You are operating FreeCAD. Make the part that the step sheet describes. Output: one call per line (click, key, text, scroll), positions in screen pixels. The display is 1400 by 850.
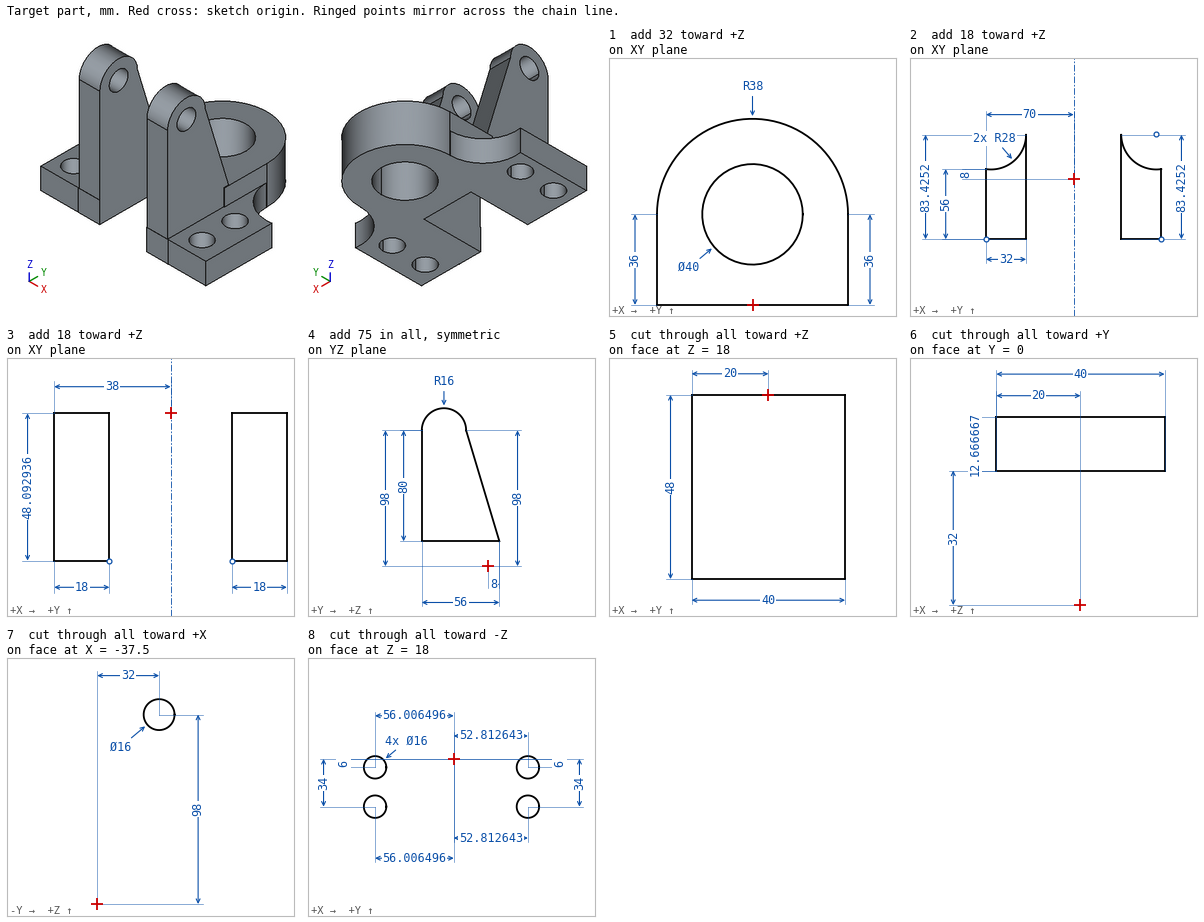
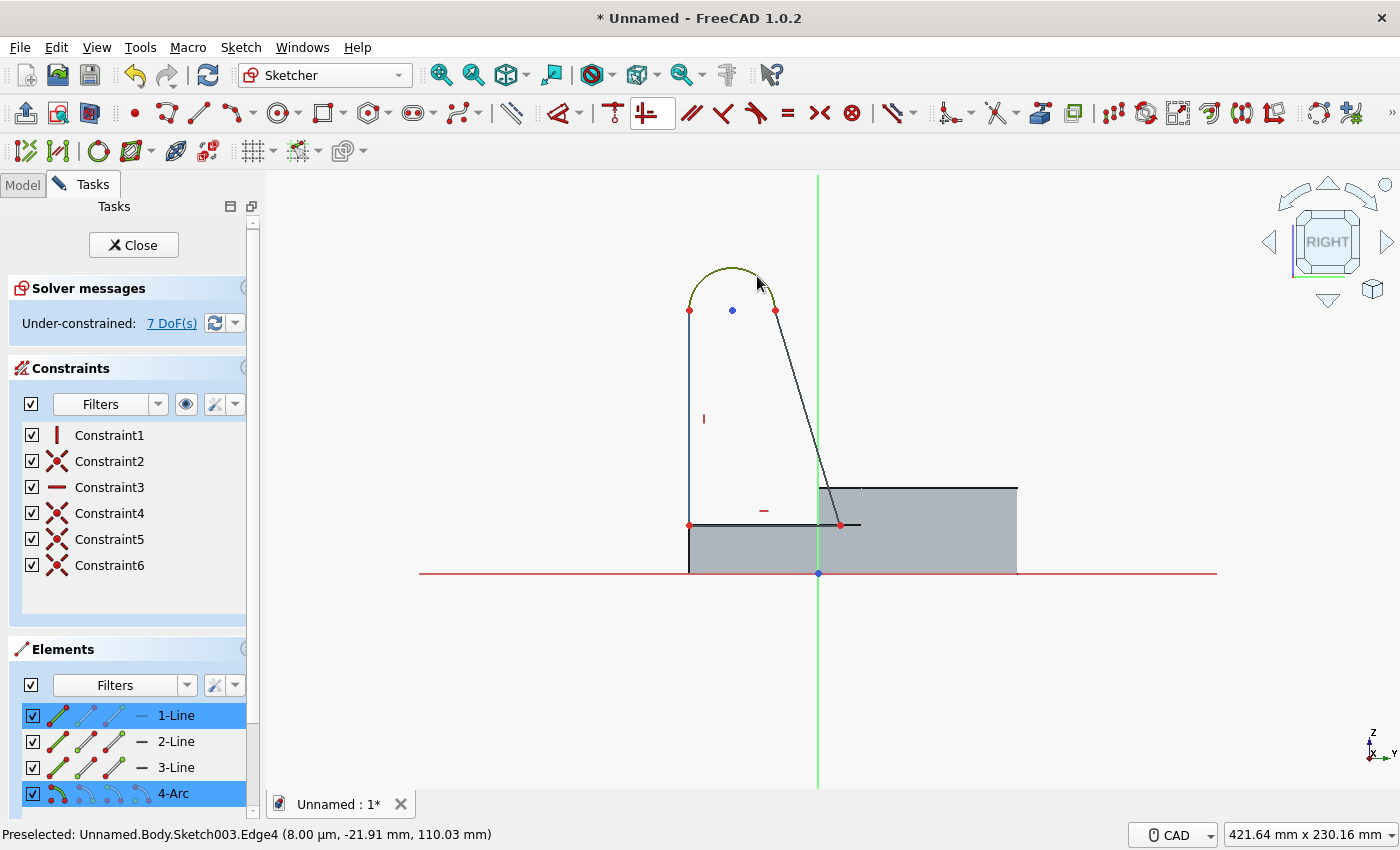
click(756, 114)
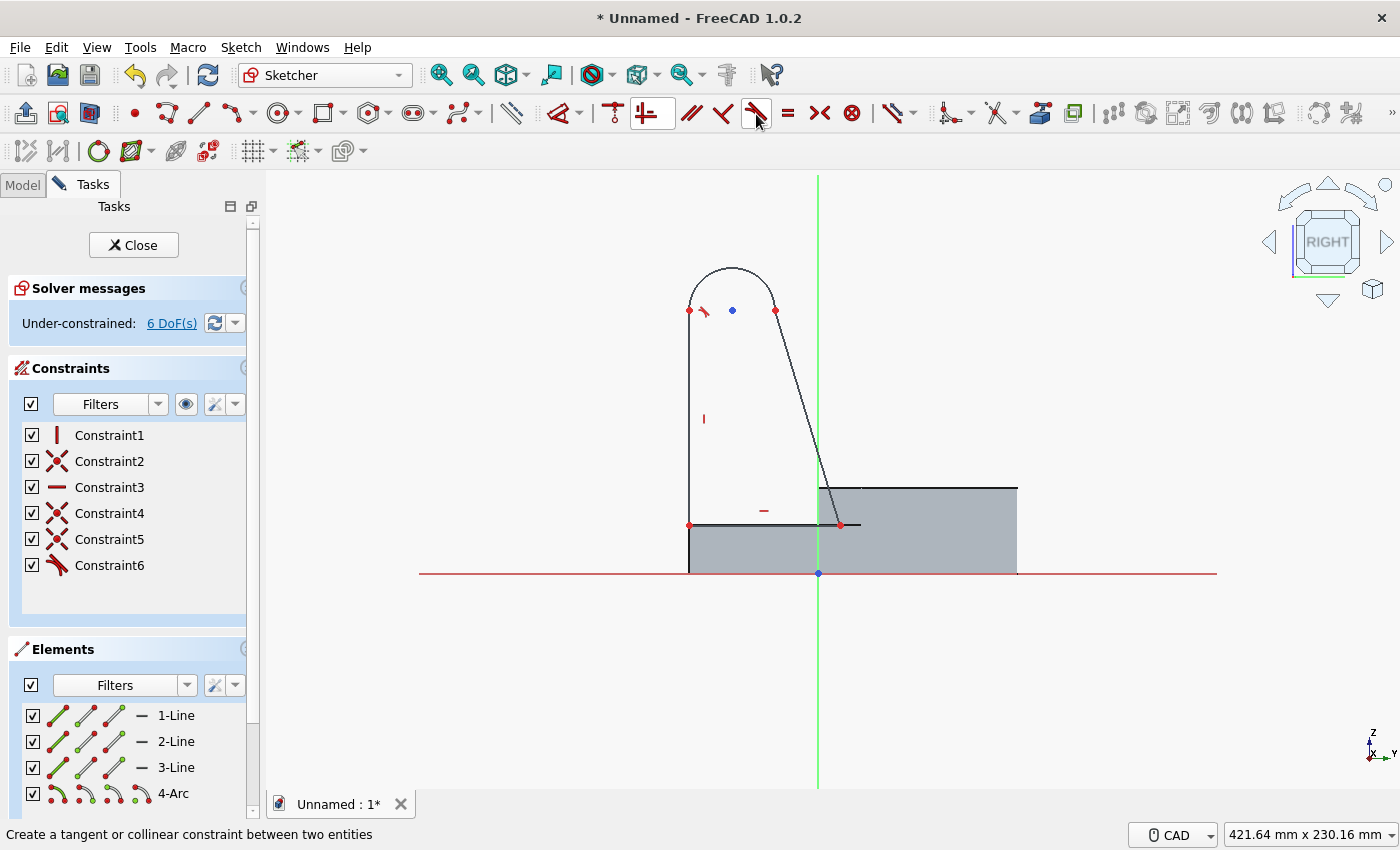
click(558, 114)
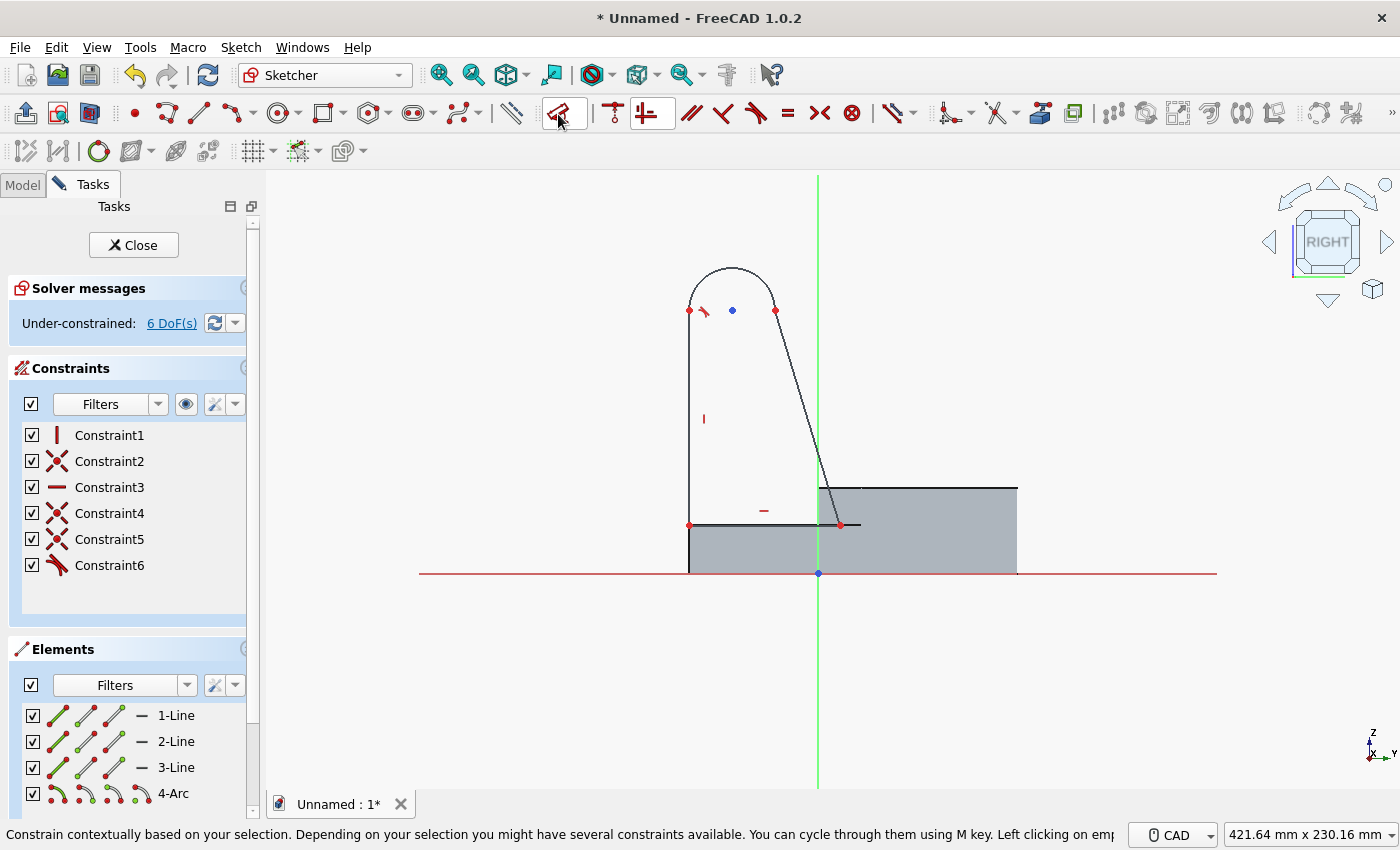
click(757, 276)
click(776, 250)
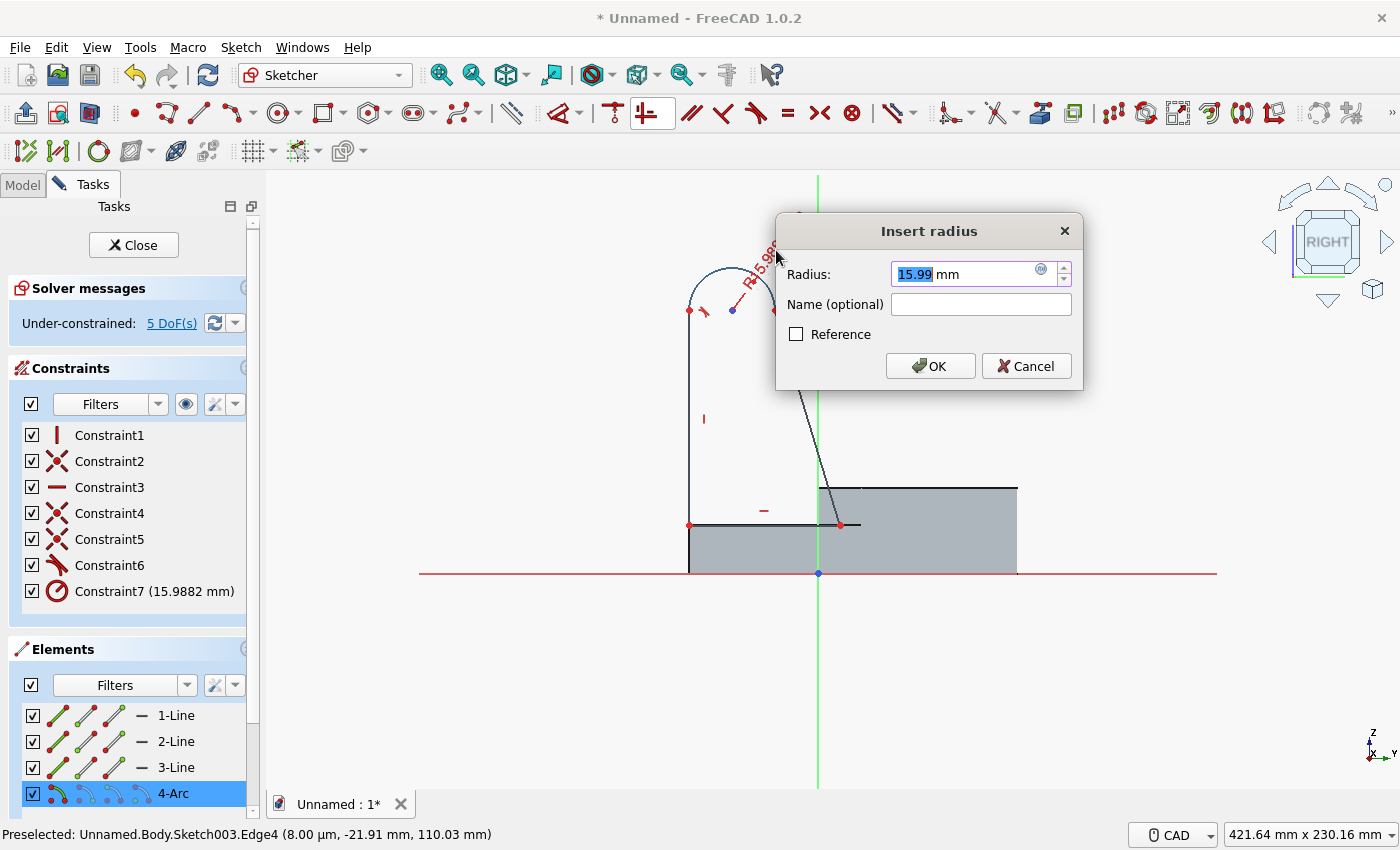
text(16)
key(Return)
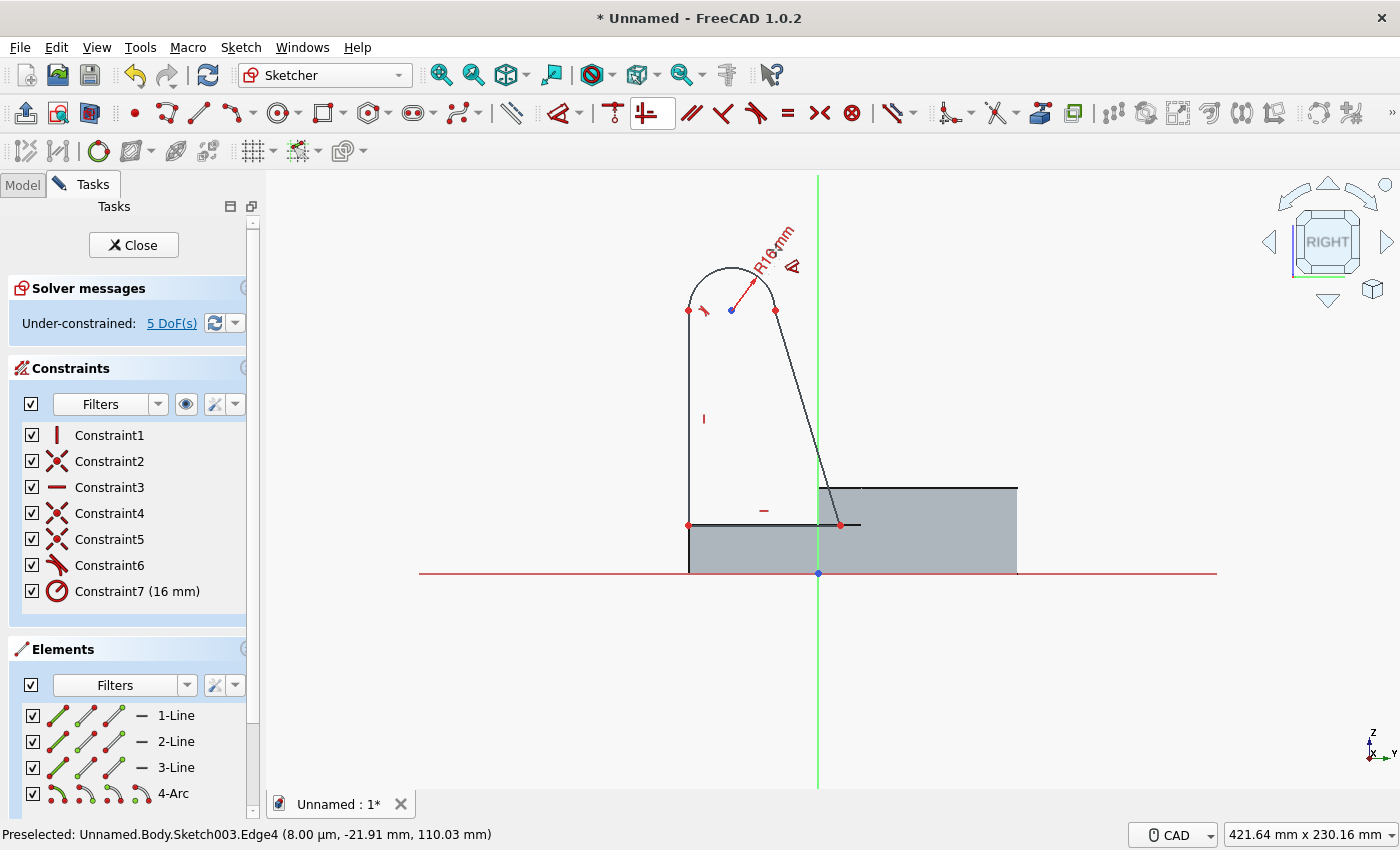
click(689, 376)
click(655, 419)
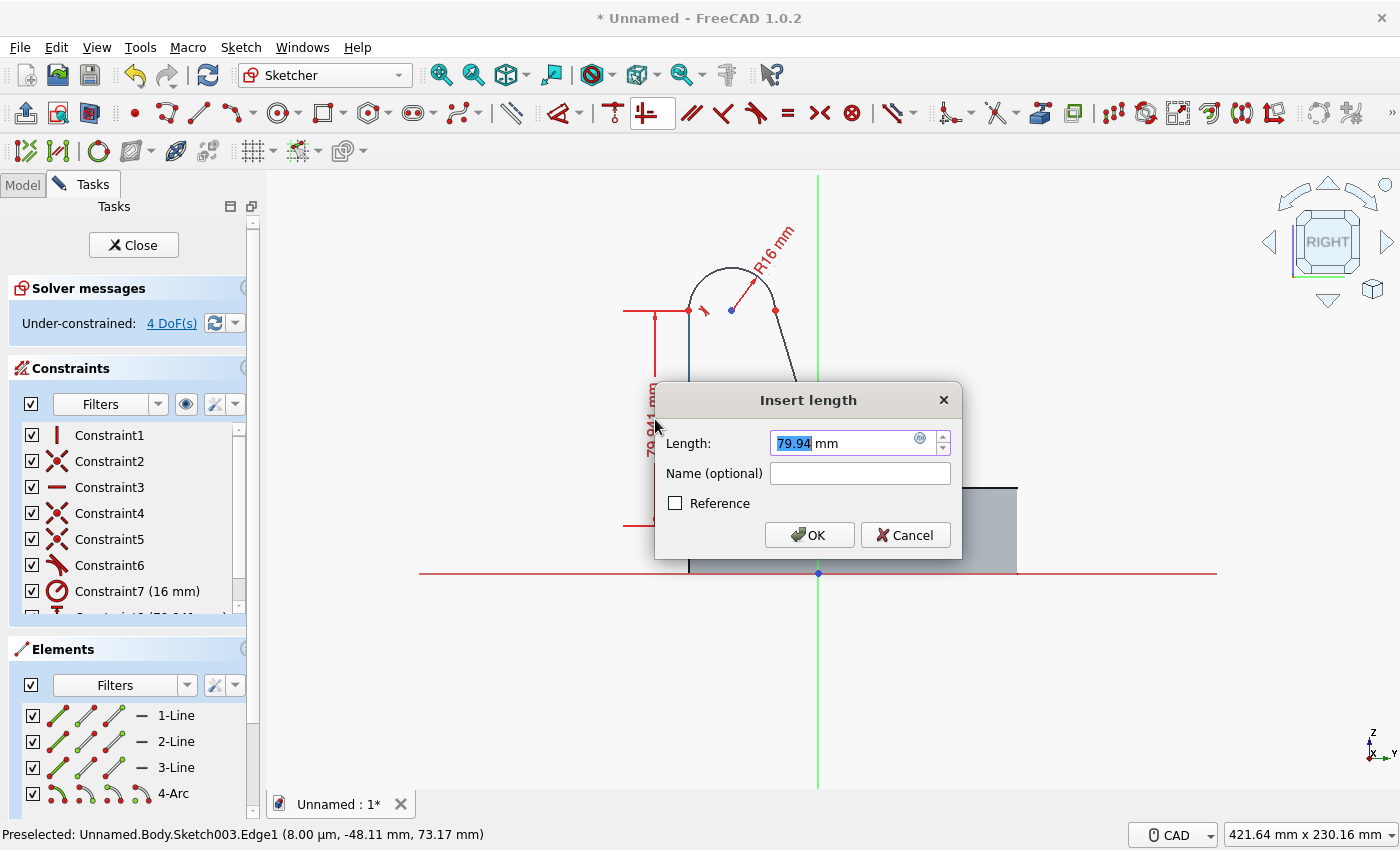
text(80)
key(Return)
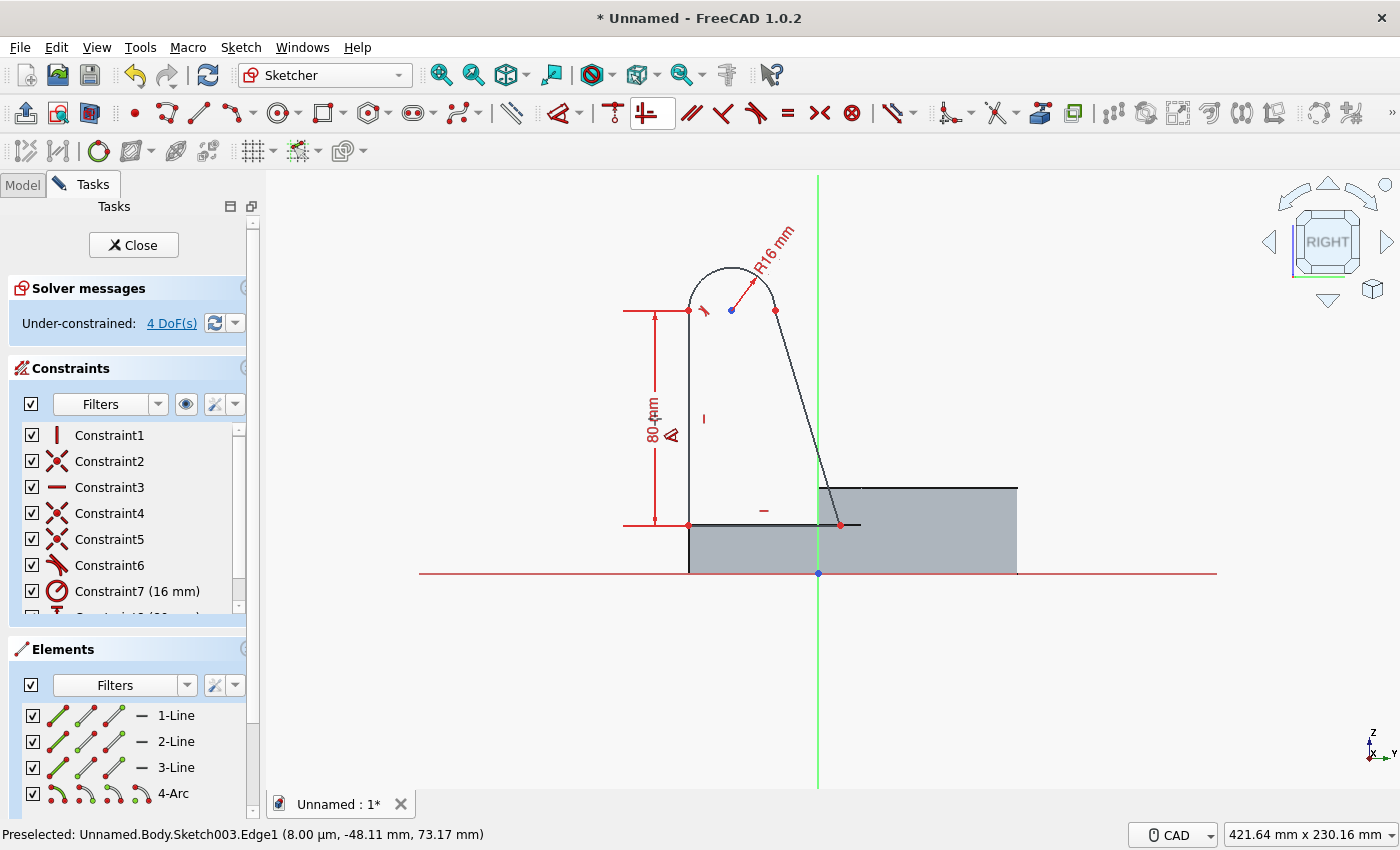
click(734, 526)
click(764, 560)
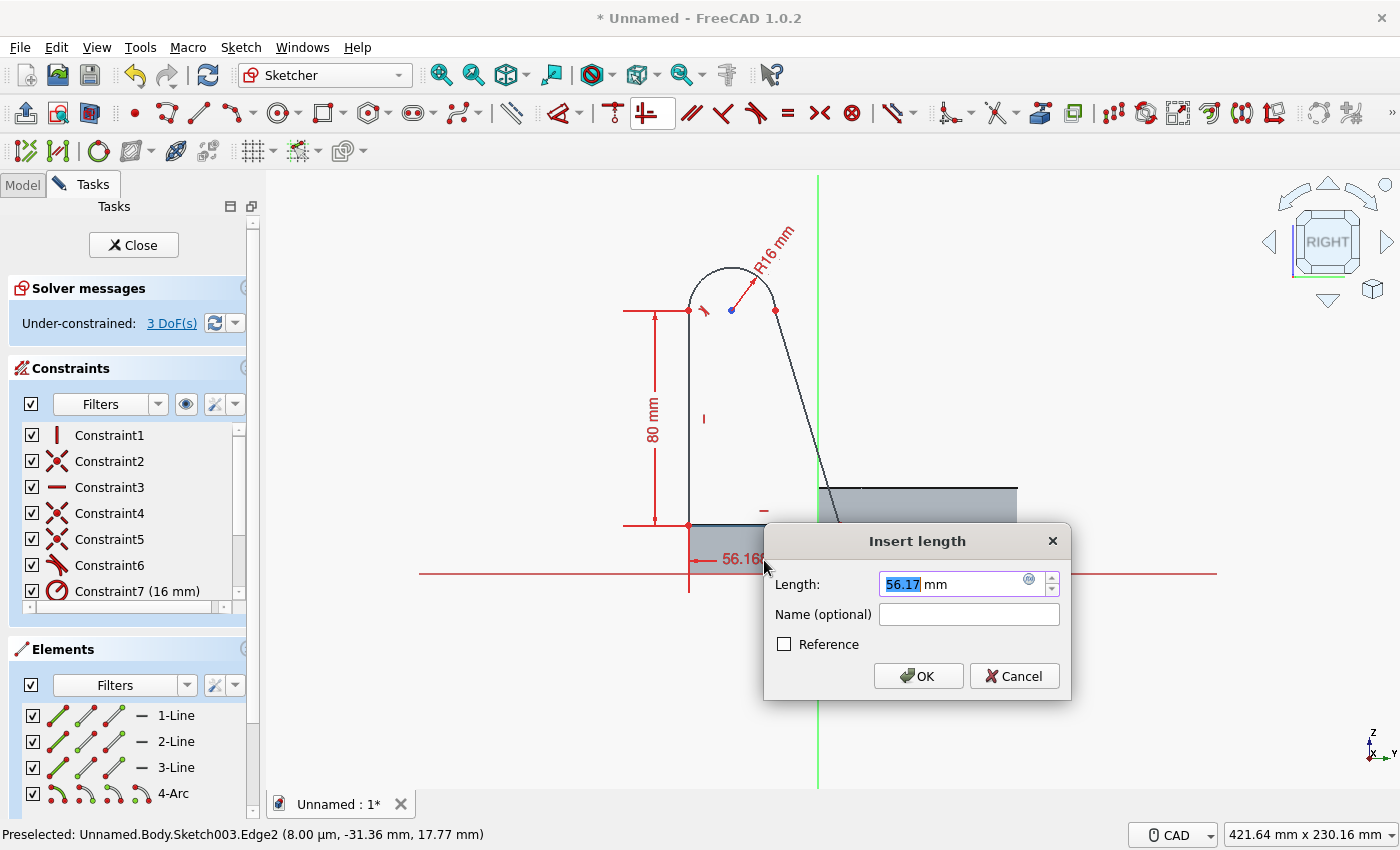
text(56)
key(Return)